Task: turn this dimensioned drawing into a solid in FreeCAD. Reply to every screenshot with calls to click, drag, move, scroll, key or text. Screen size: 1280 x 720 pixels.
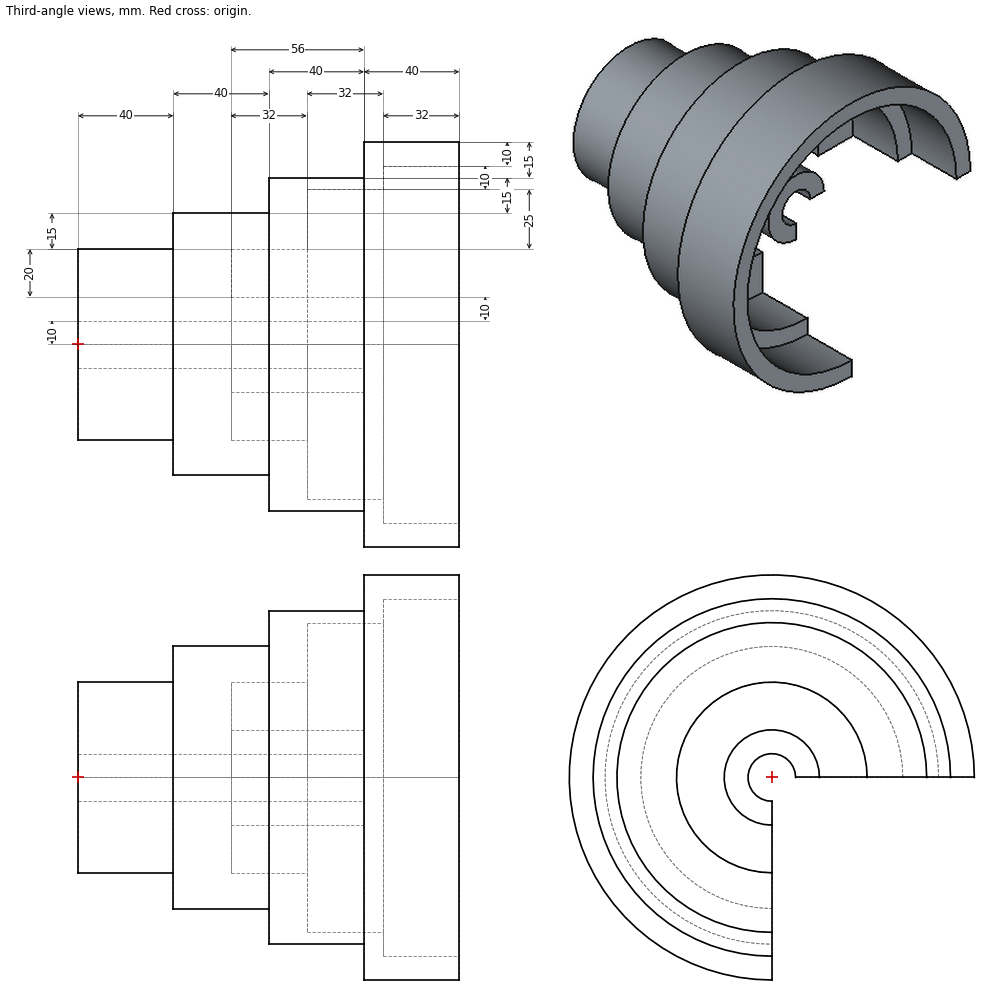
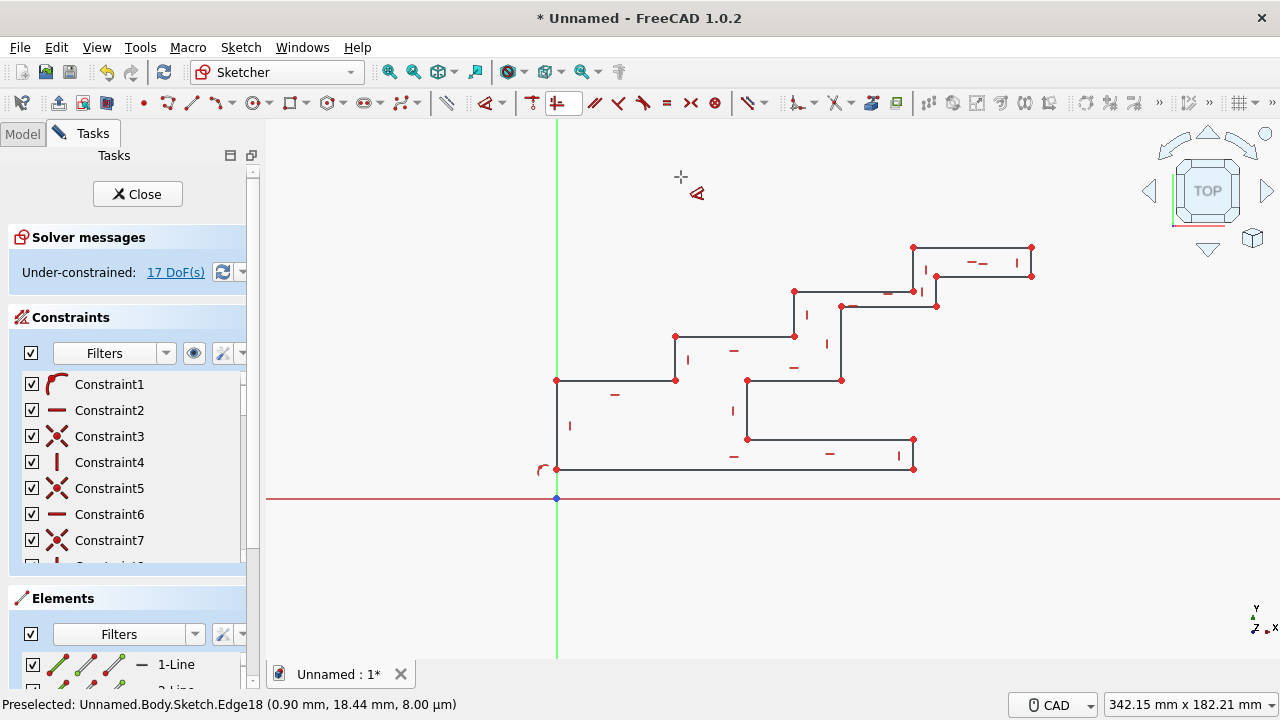
scroll(913, 458, up, 2)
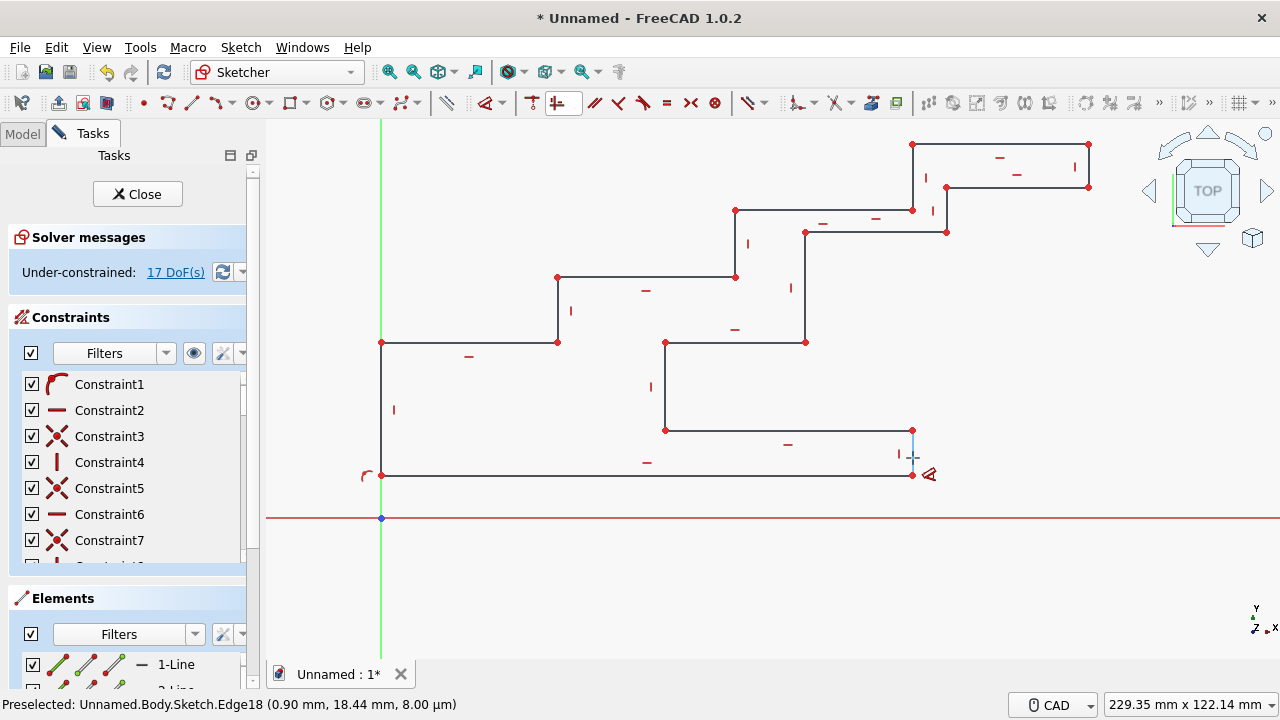
click(913, 458)
click(947, 453)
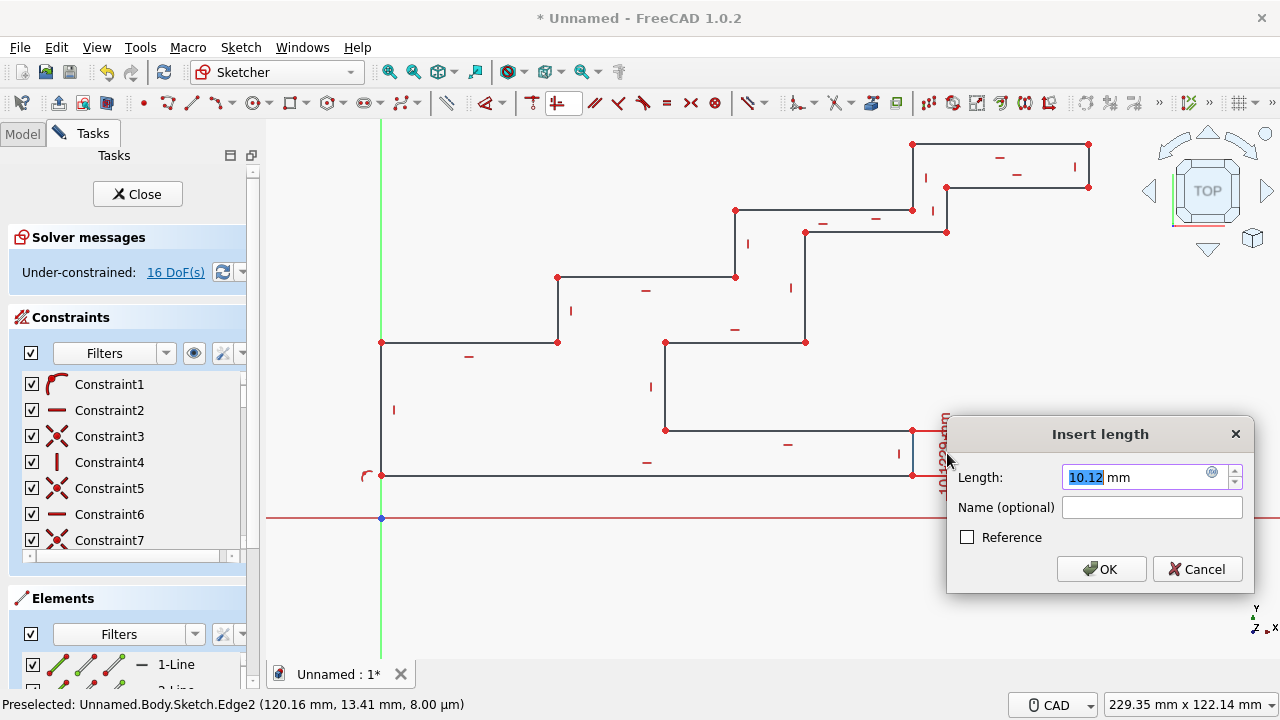
text(10)
key(Return)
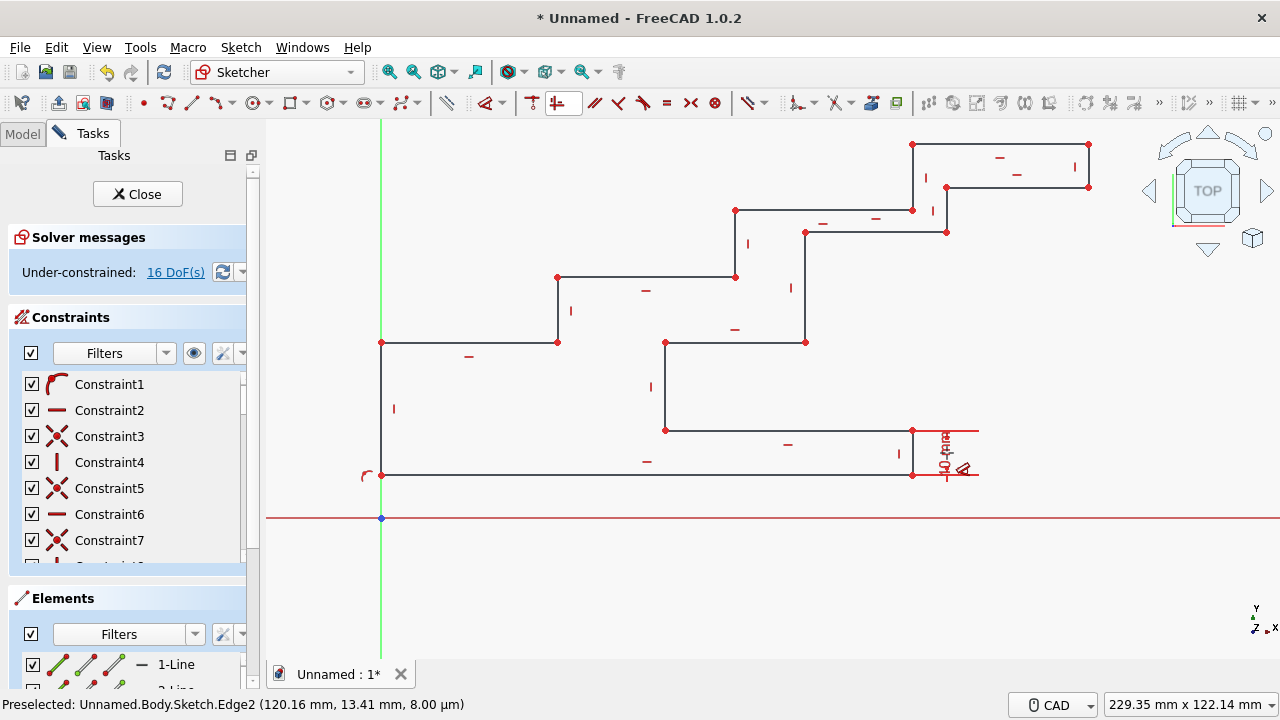
click(838, 431)
click(789, 397)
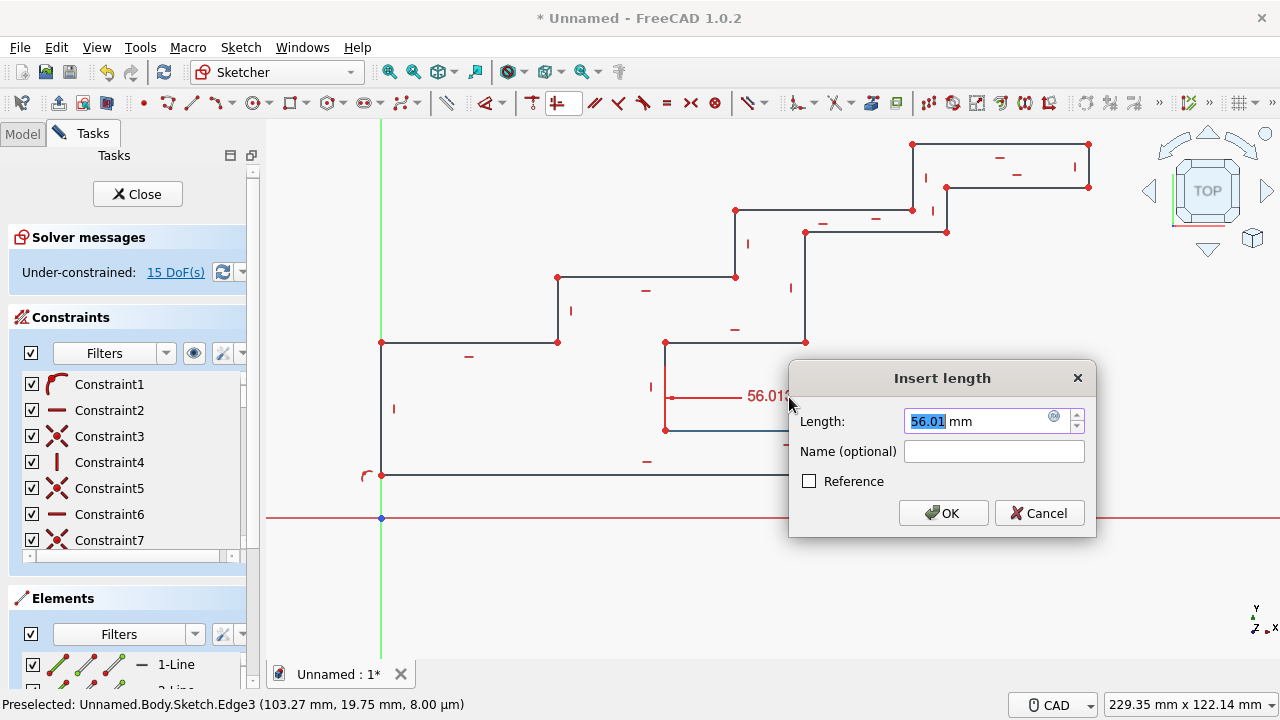
text(56)
key(Return)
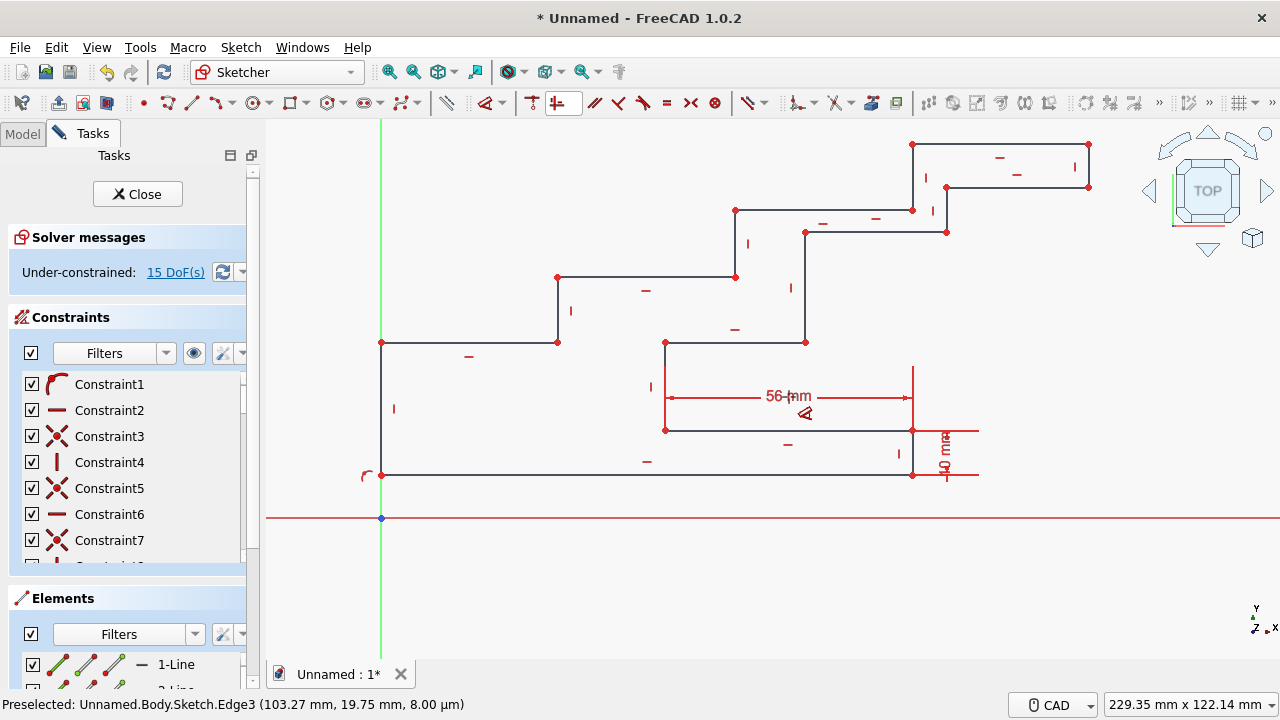
click(665, 405)
click(631, 387)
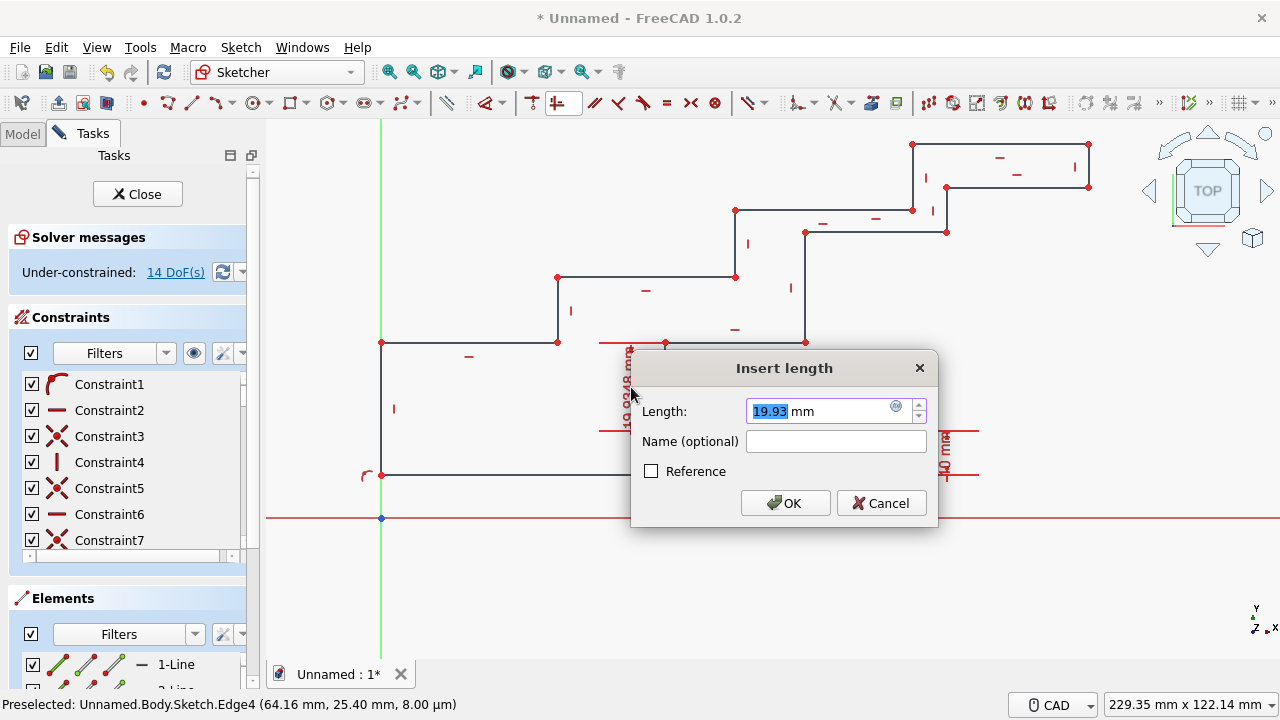
text(20)
key(Return)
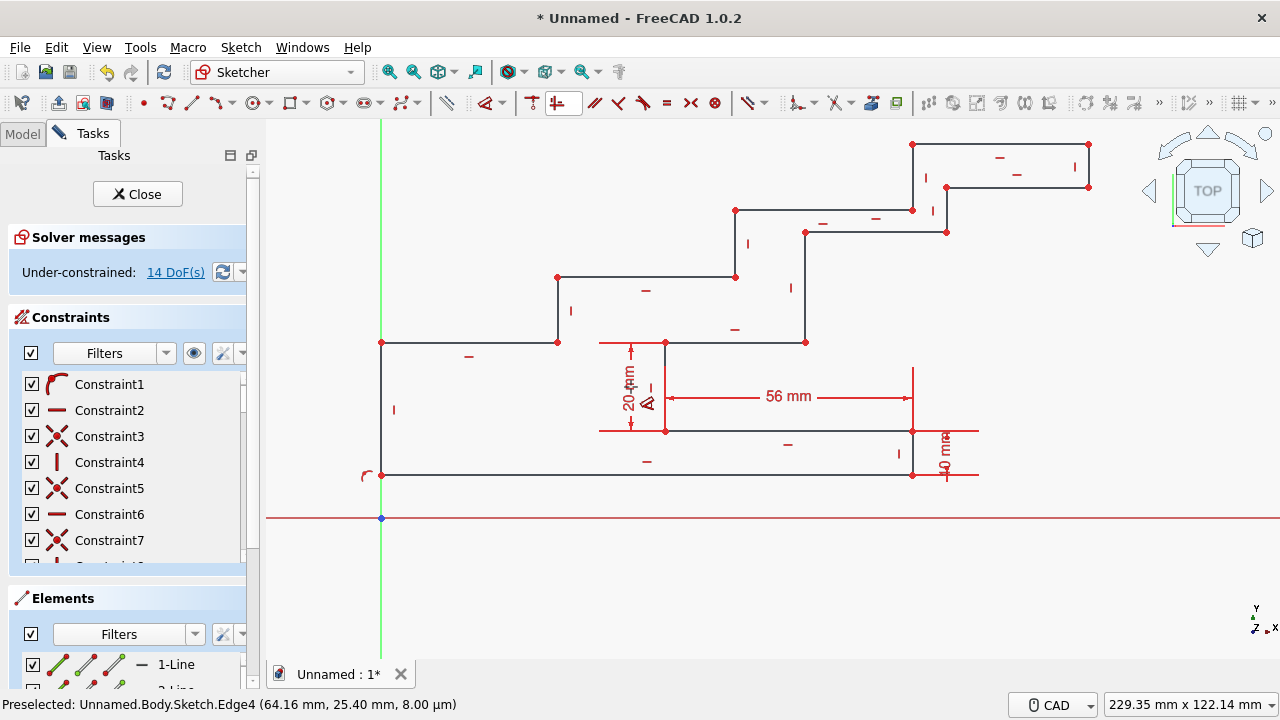
click(707, 343)
click(735, 377)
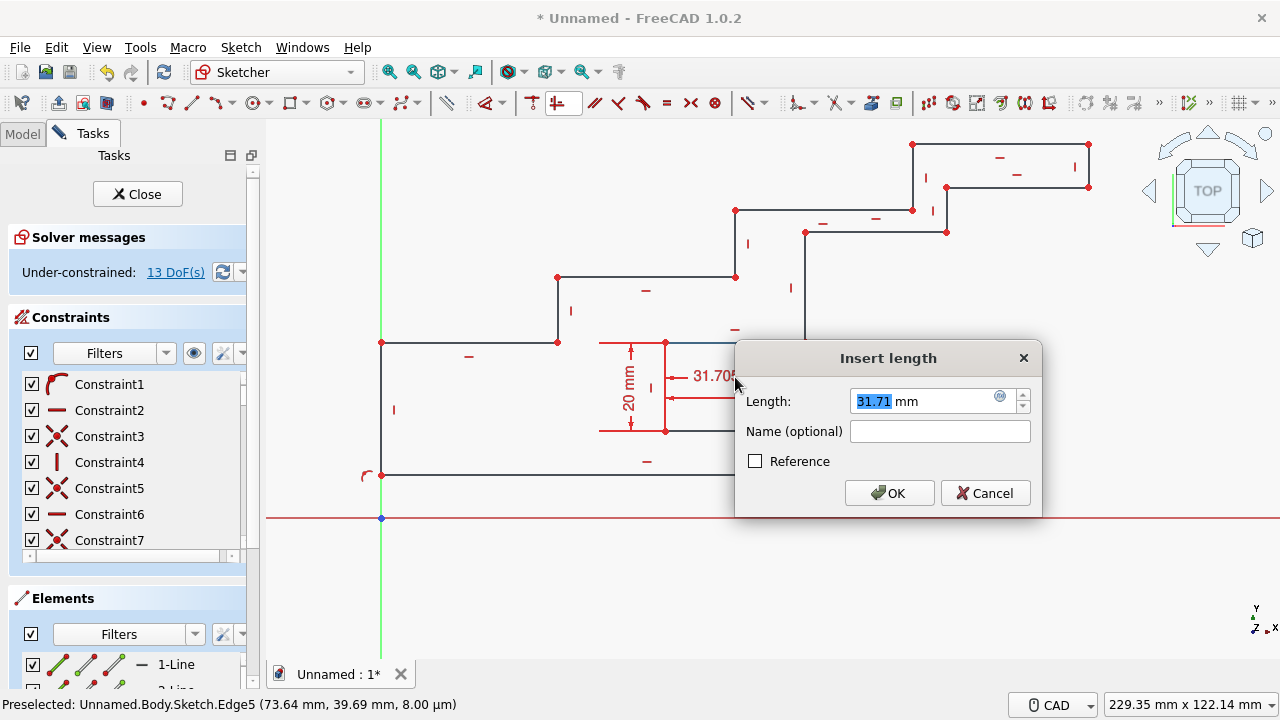
text(32)
key(Return)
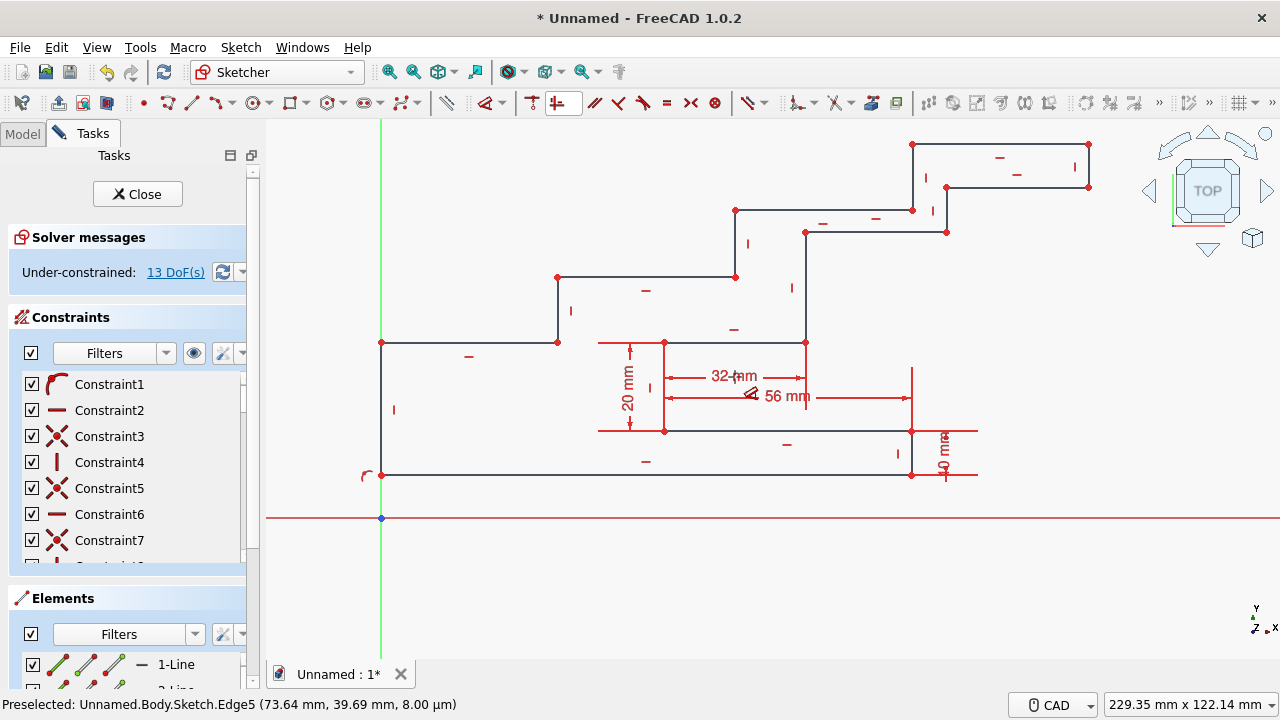
click(806, 310)
click(840, 288)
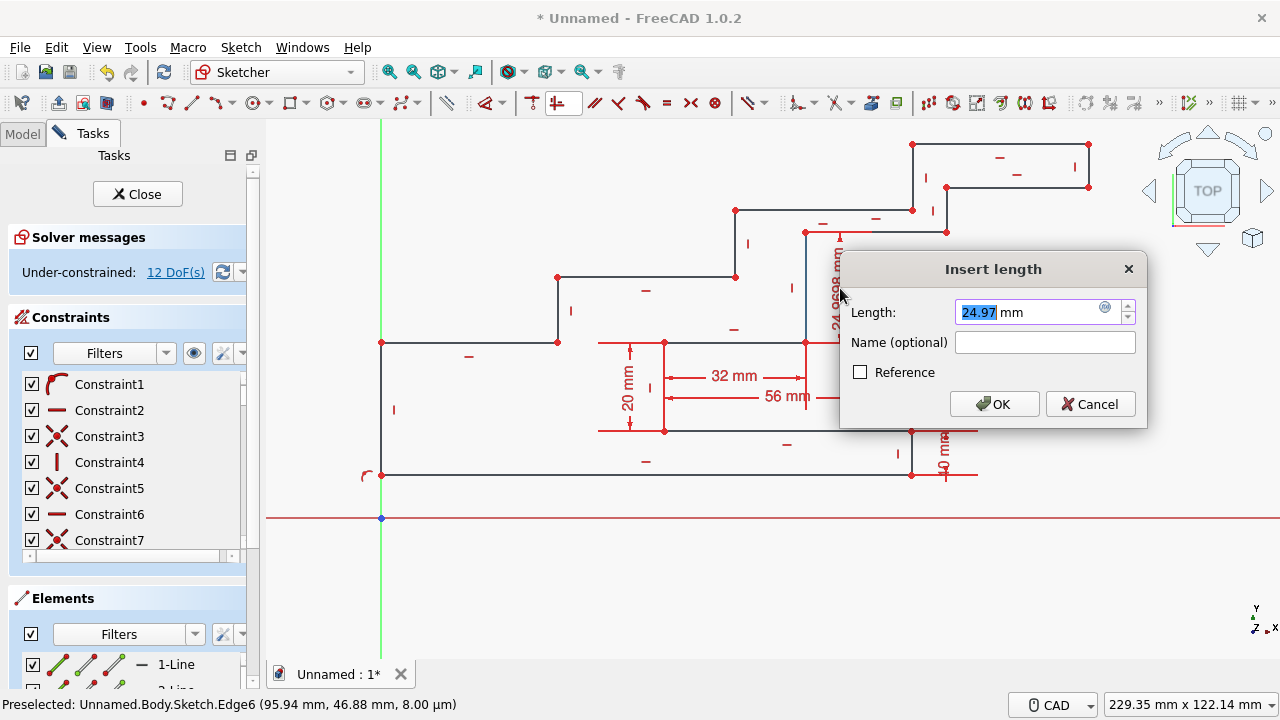
text(25)
key(Return)